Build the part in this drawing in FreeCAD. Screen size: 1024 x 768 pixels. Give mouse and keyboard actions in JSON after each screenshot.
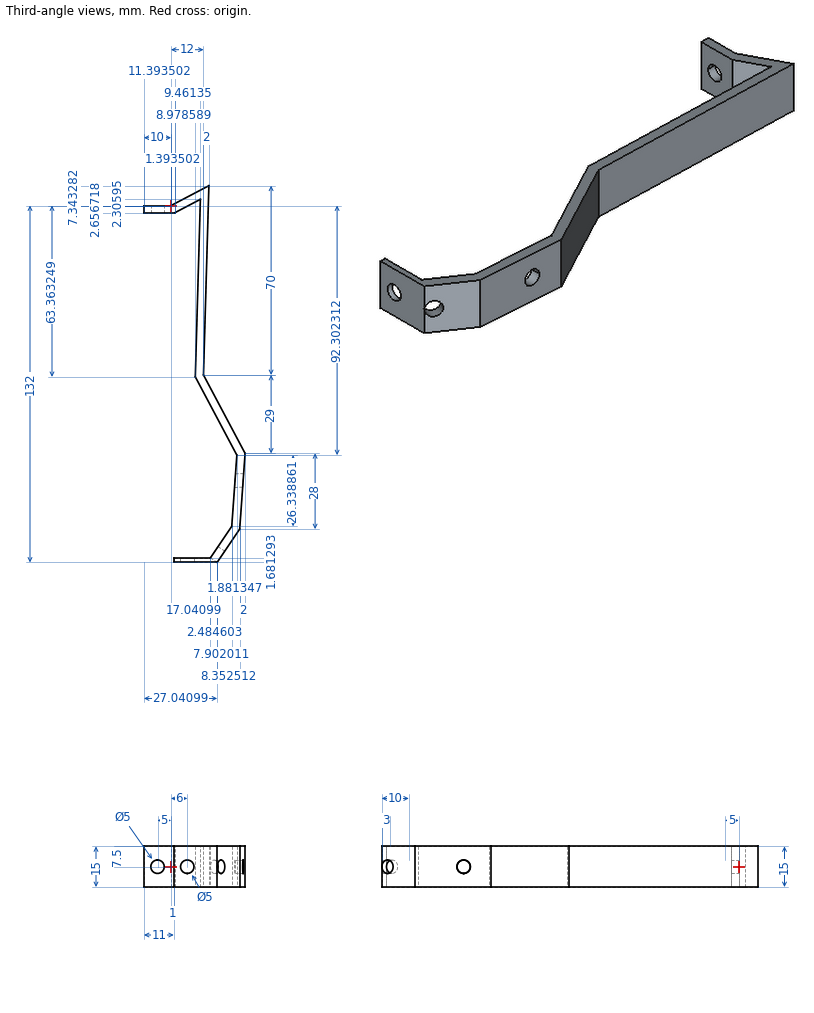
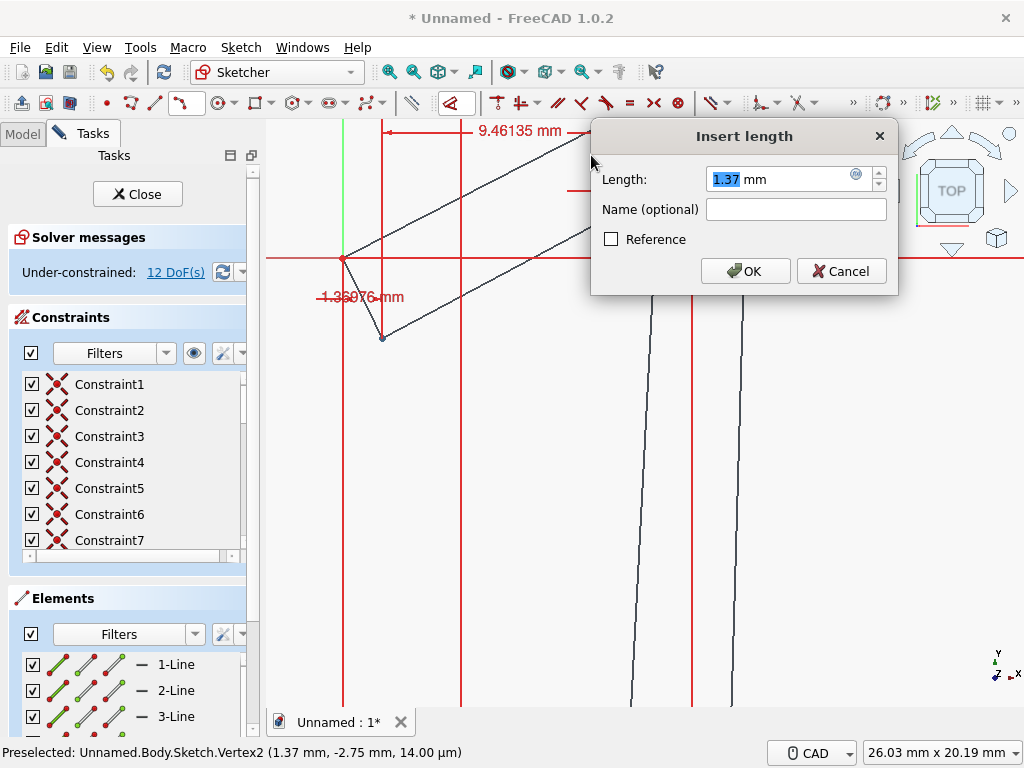
{"action": "type", "text": "1.393502"}
{"action": "key", "text": "Return"}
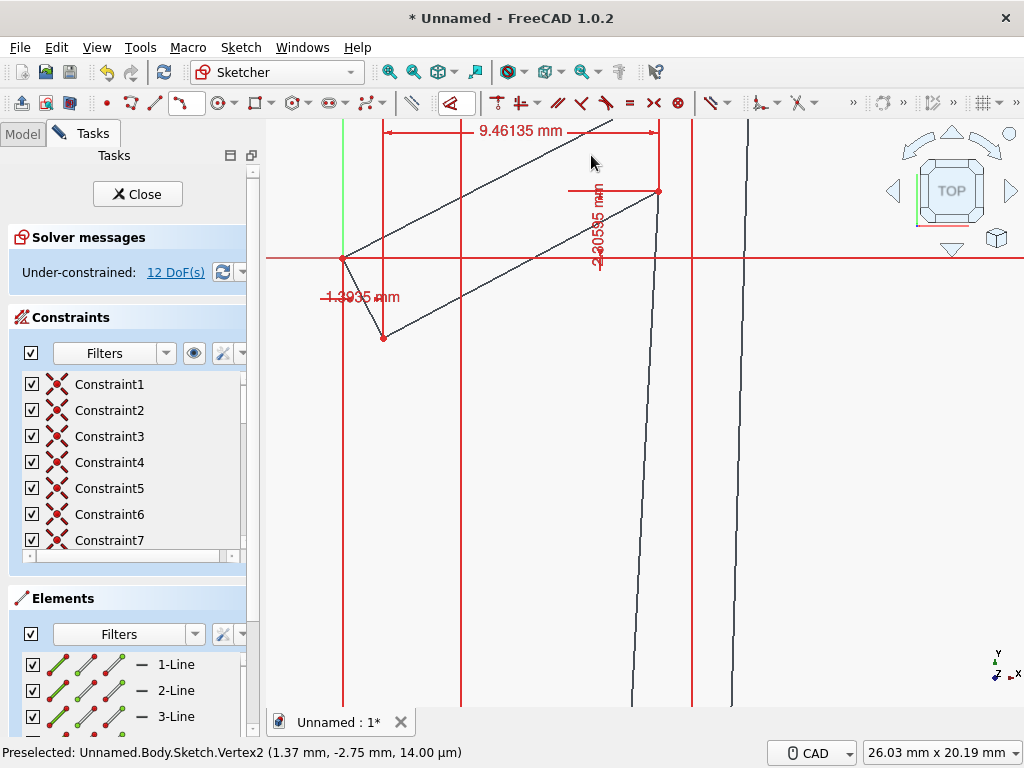
{"action": "left_click", "coordinate": [383, 338]}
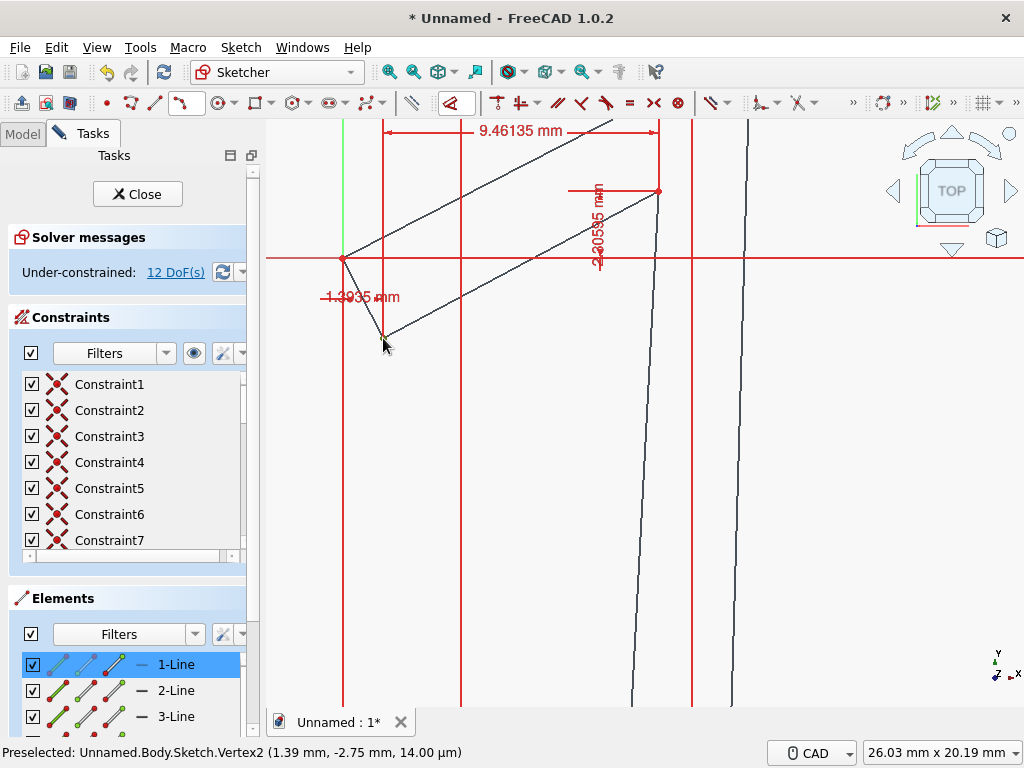
{"action": "key", "text": "i"}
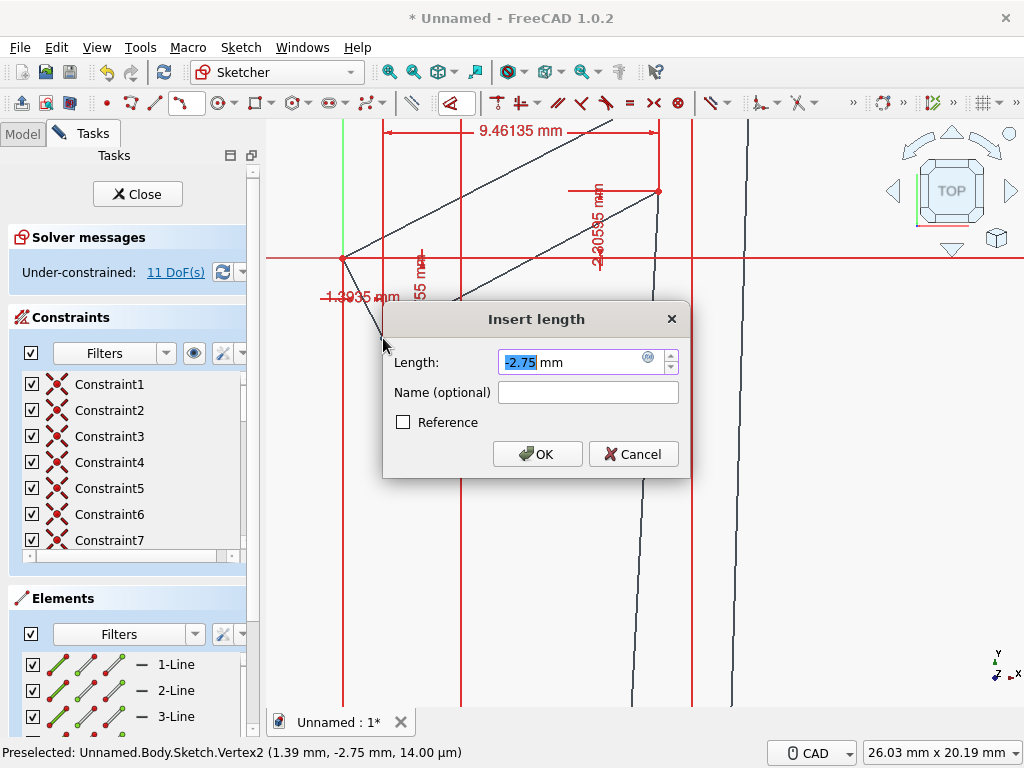
{"action": "type", "text": "-2.656718"}
{"action": "key", "text": "Return"}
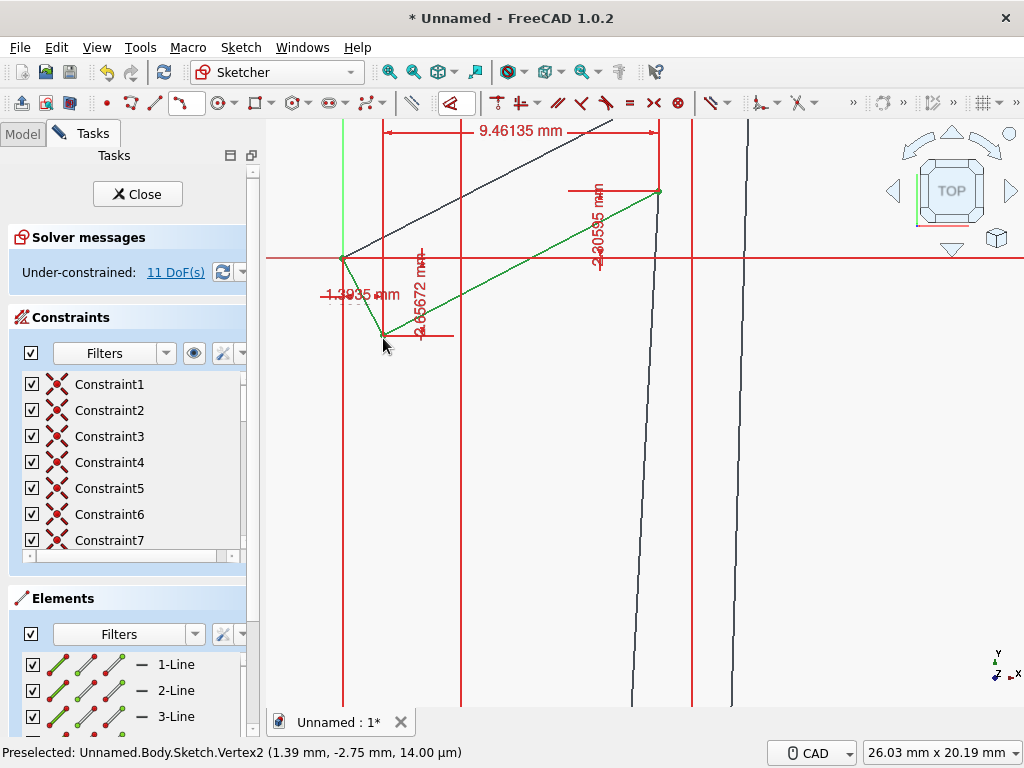
{"action": "scroll", "coordinate": [560, 247], "scroll_direction": "down", "scroll_amount": 12}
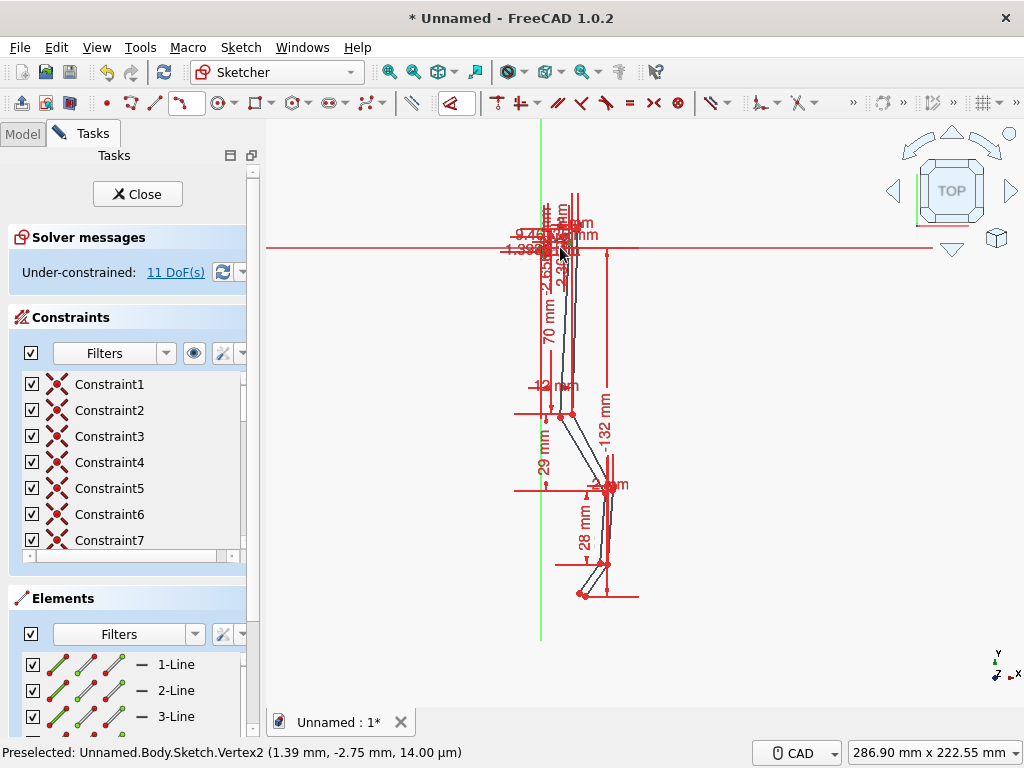
{"action": "scroll", "coordinate": [560, 417], "scroll_direction": "up", "scroll_amount": 3}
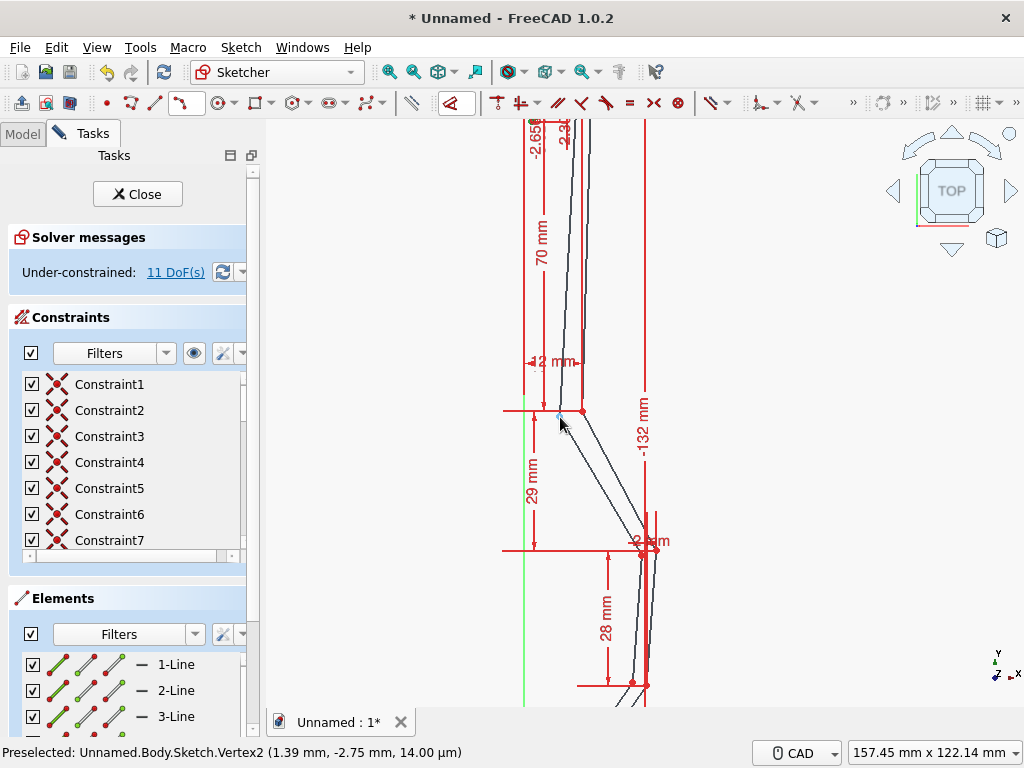
{"action": "left_click", "coordinate": [560, 417]}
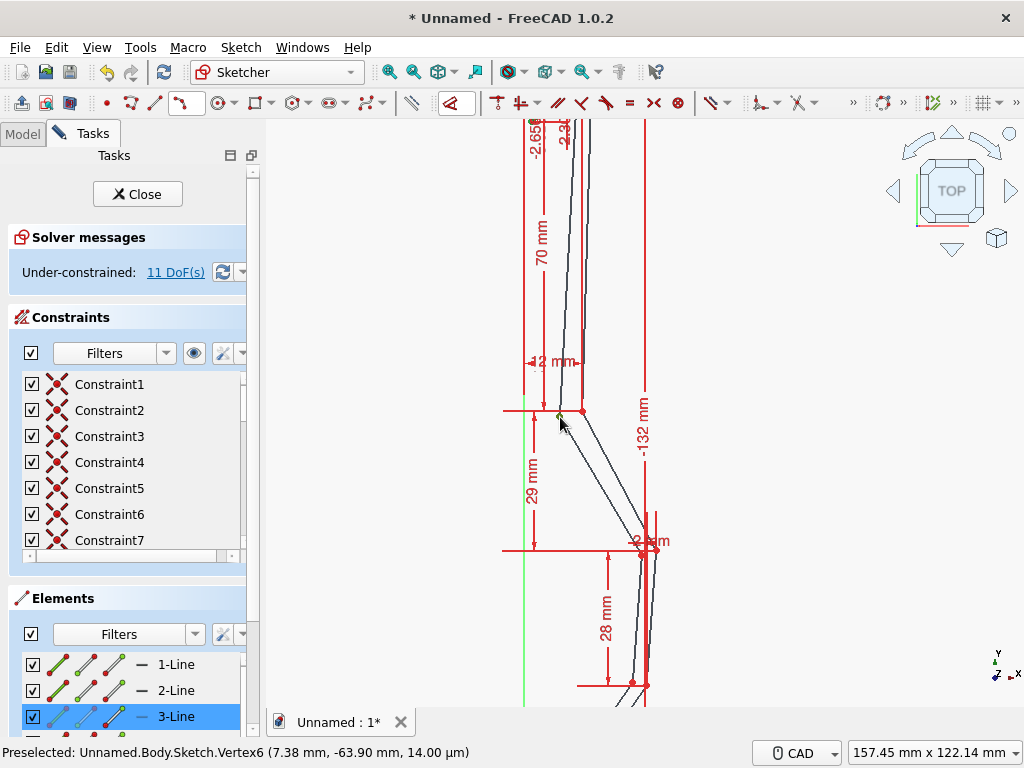
{"action": "key", "text": "l"}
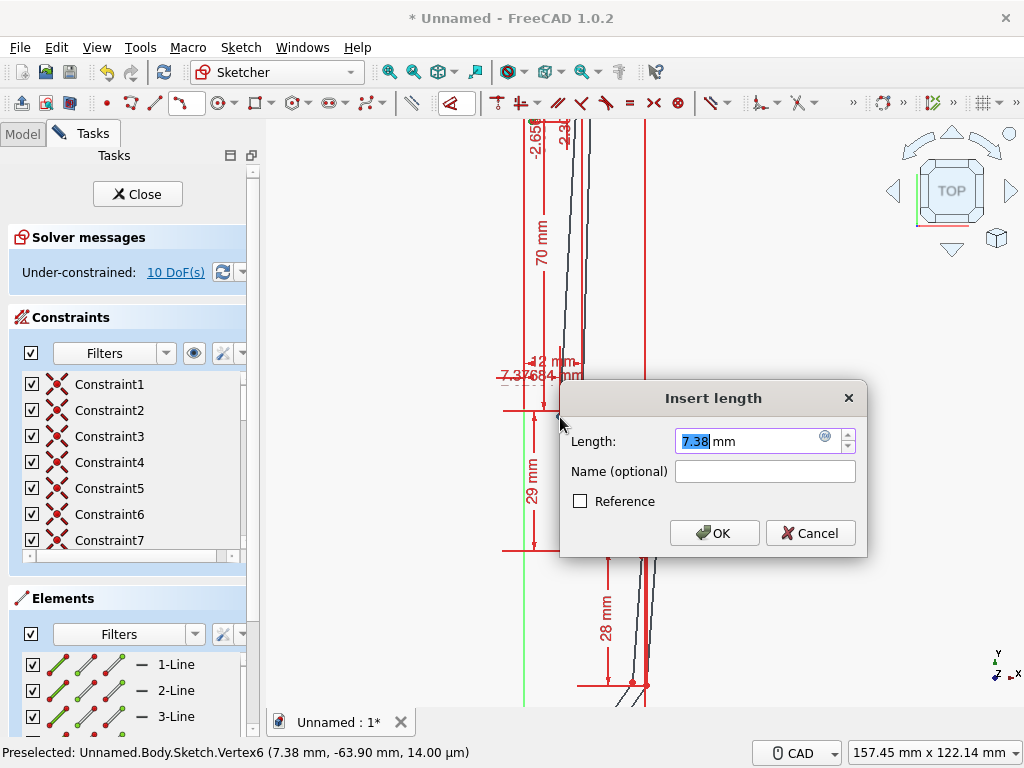
{"action": "type", "text": "8.978589"}
{"action": "key", "text": "Return"}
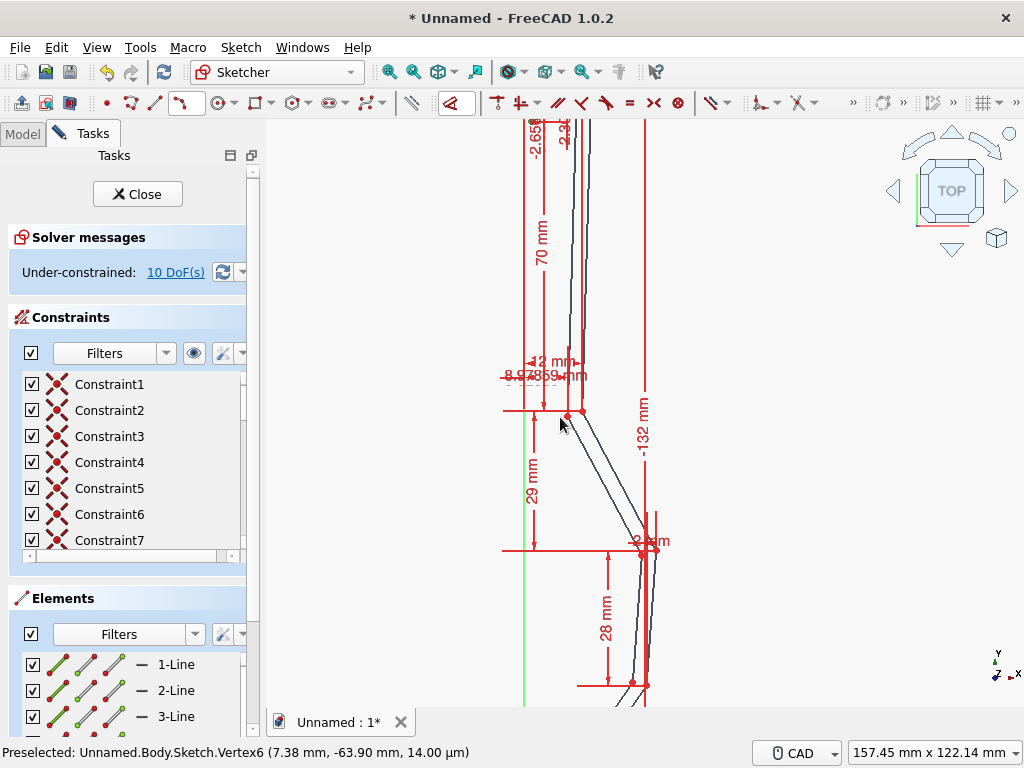
{"action": "scroll", "coordinate": [560, 418], "scroll_direction": "down", "scroll_amount": 3}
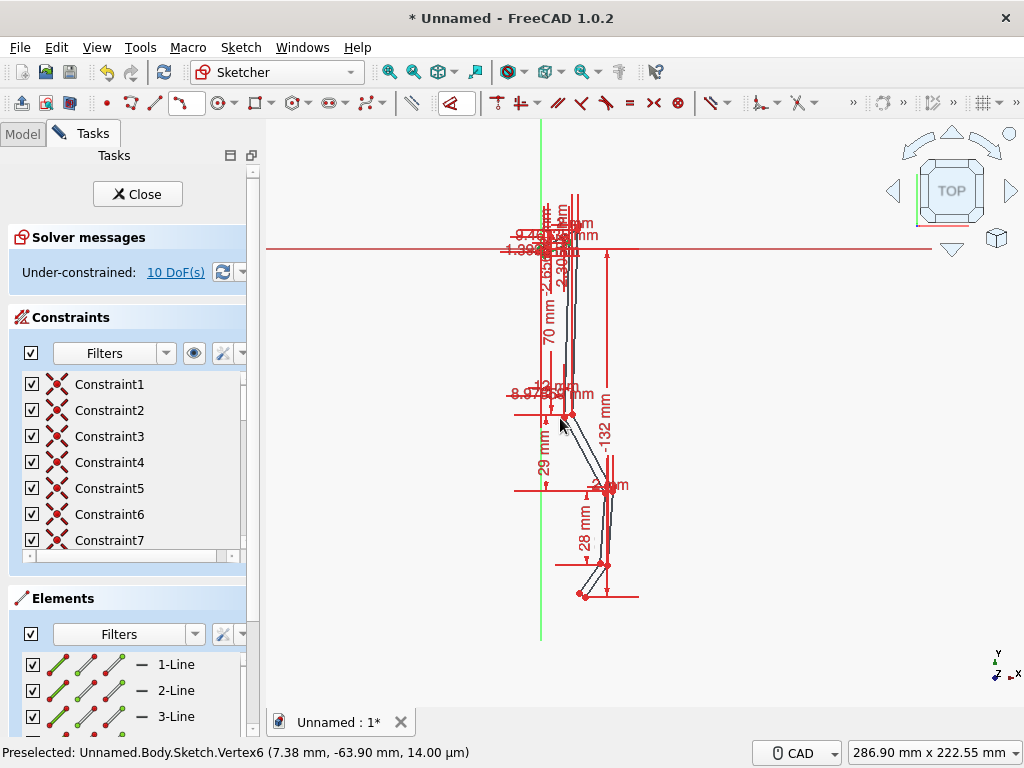
{"action": "scroll", "coordinate": [585, 597], "scroll_direction": "up", "scroll_amount": 3}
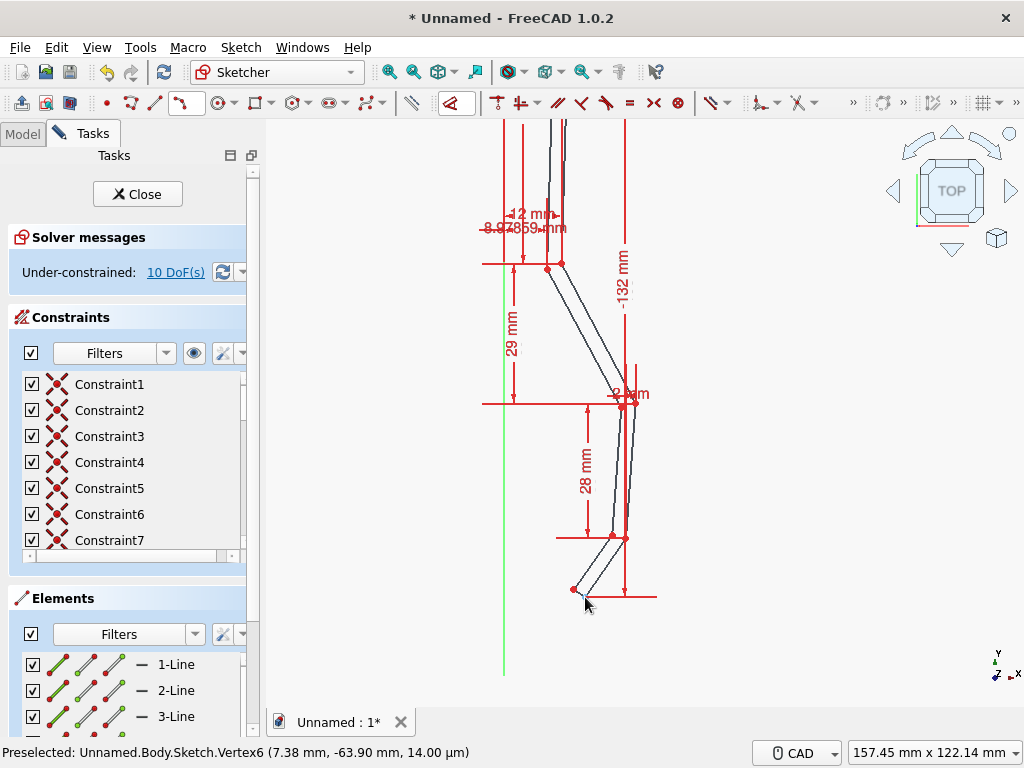
{"action": "left_click", "coordinate": [585, 597]}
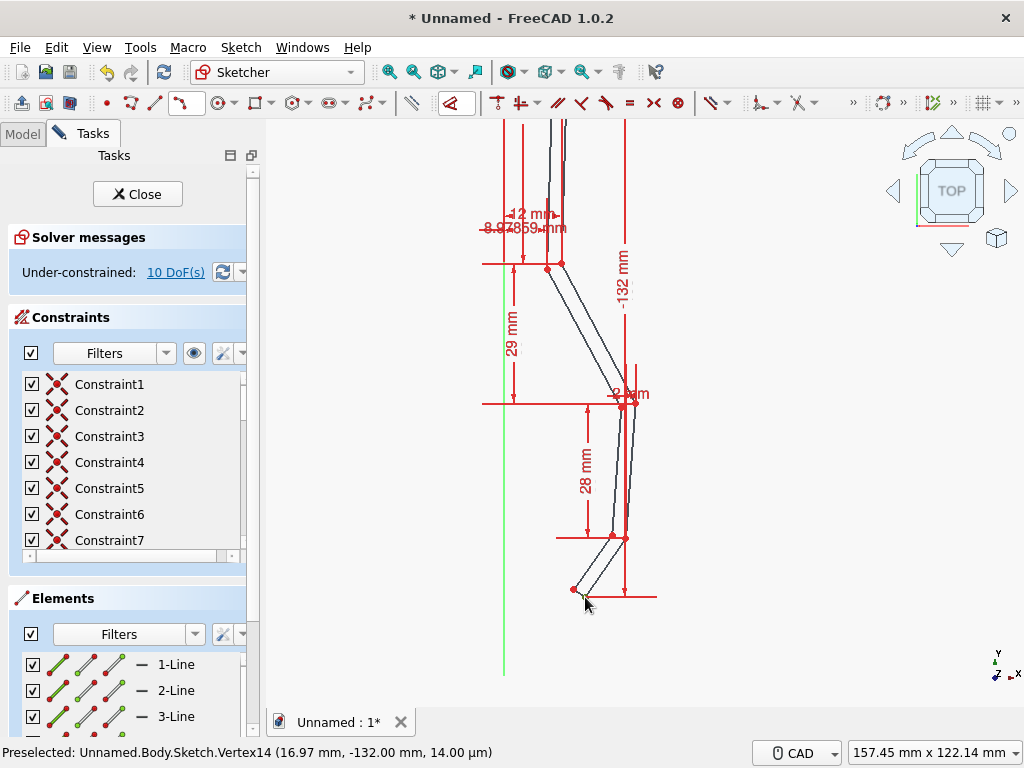
{"action": "left_click", "coordinate": [470, 104]}